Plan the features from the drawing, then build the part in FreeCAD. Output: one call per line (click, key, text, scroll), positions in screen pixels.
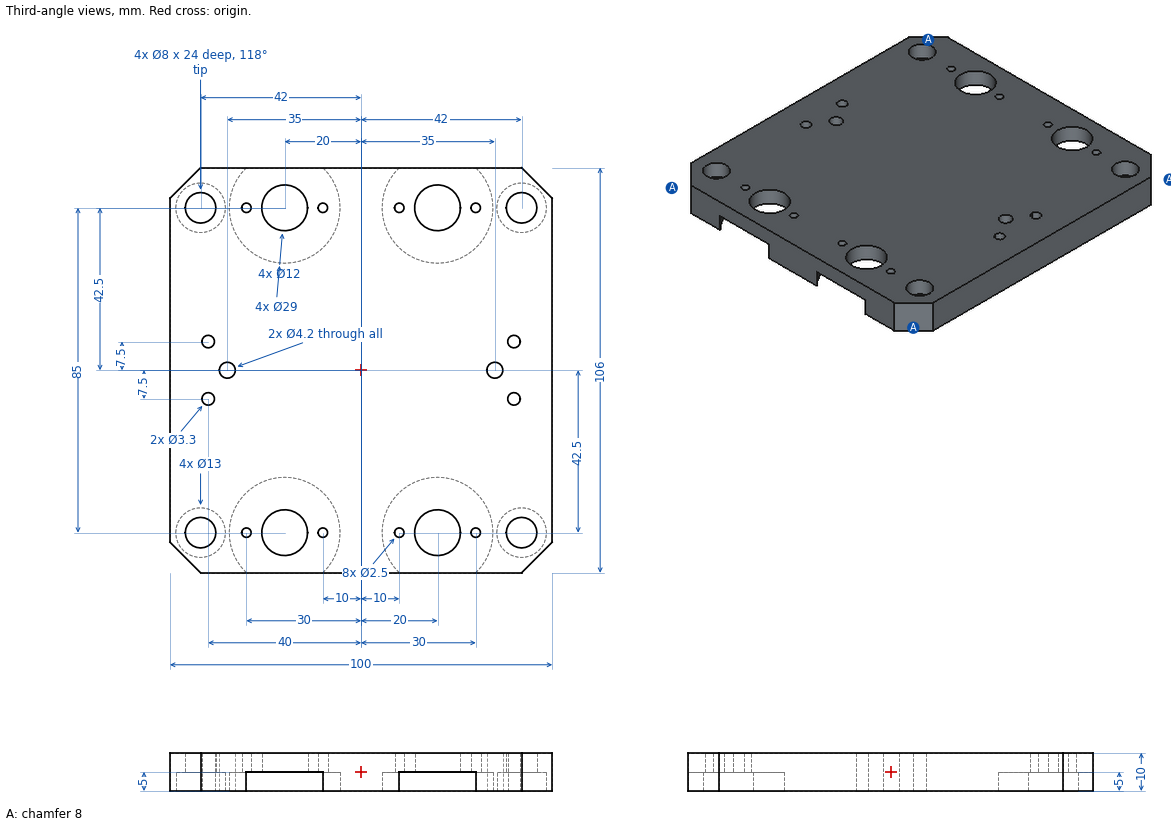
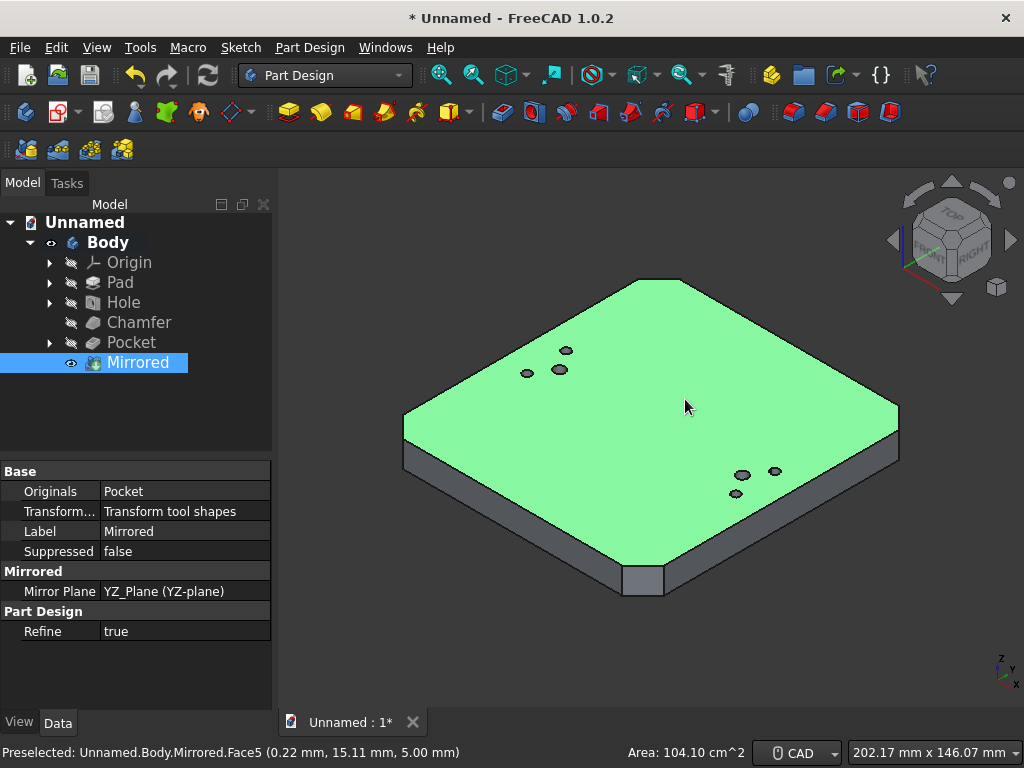
click(58, 112)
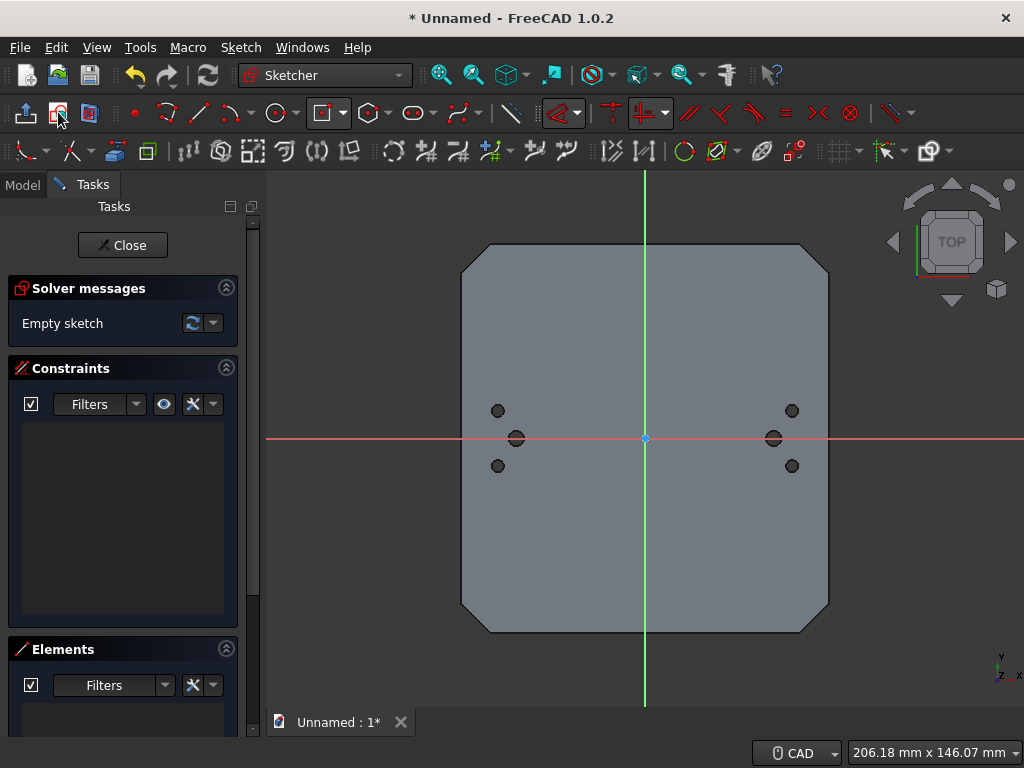
click(276, 114)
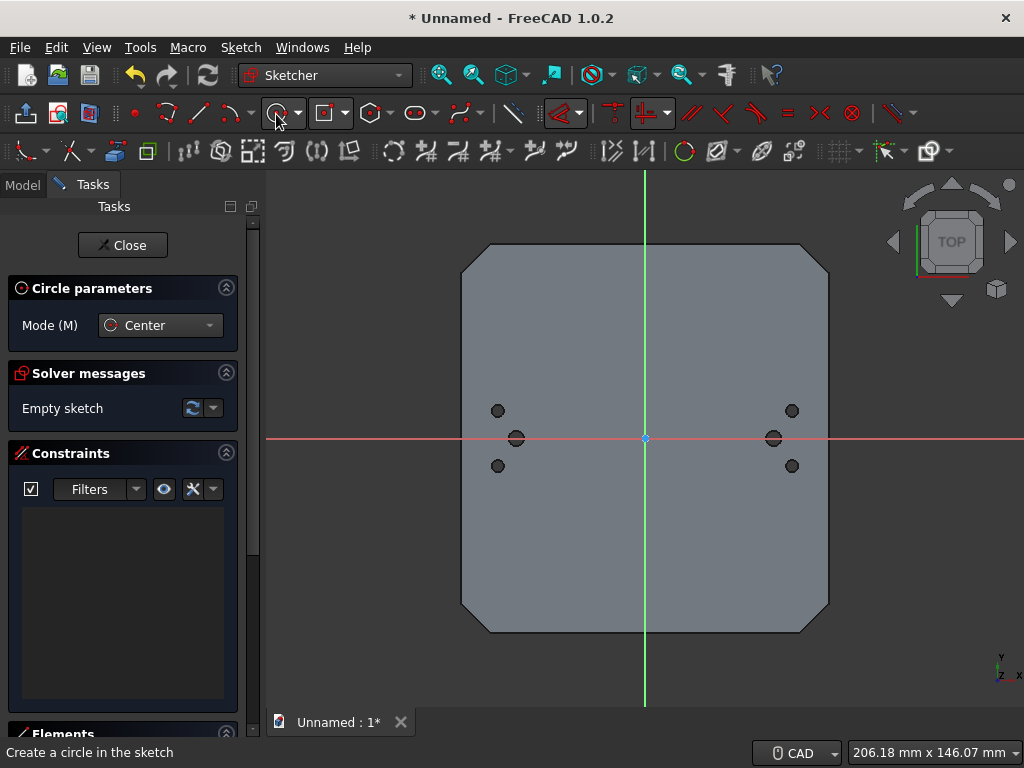
click(571, 282)
move(587, 267)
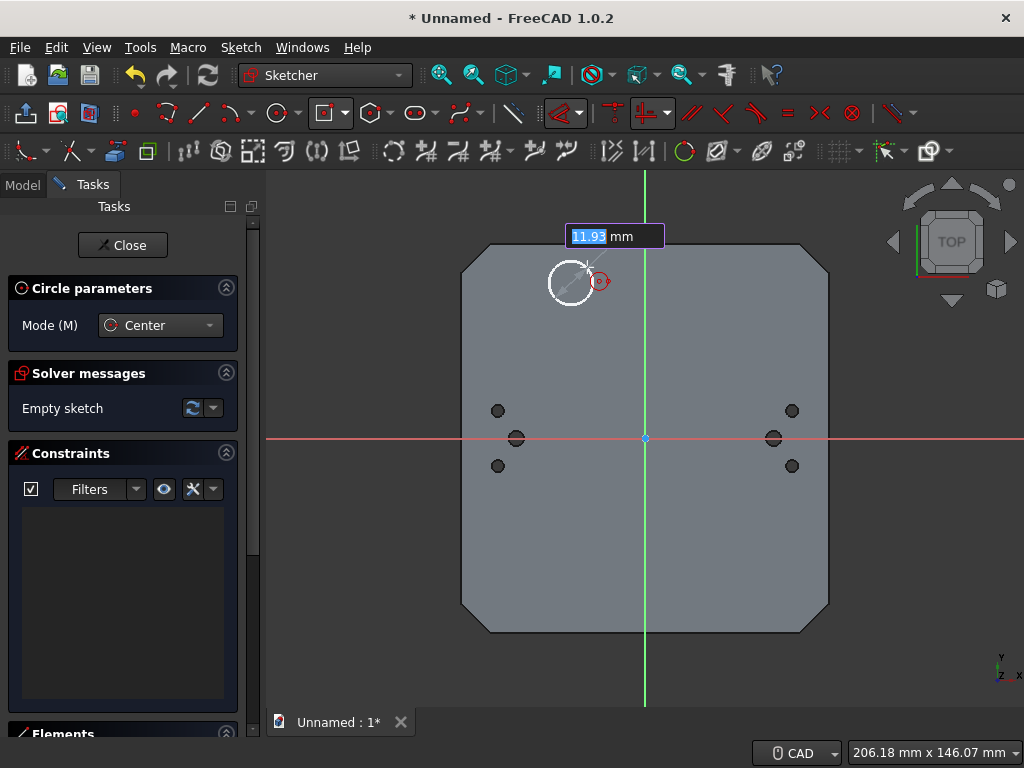
text(12)
key(Return)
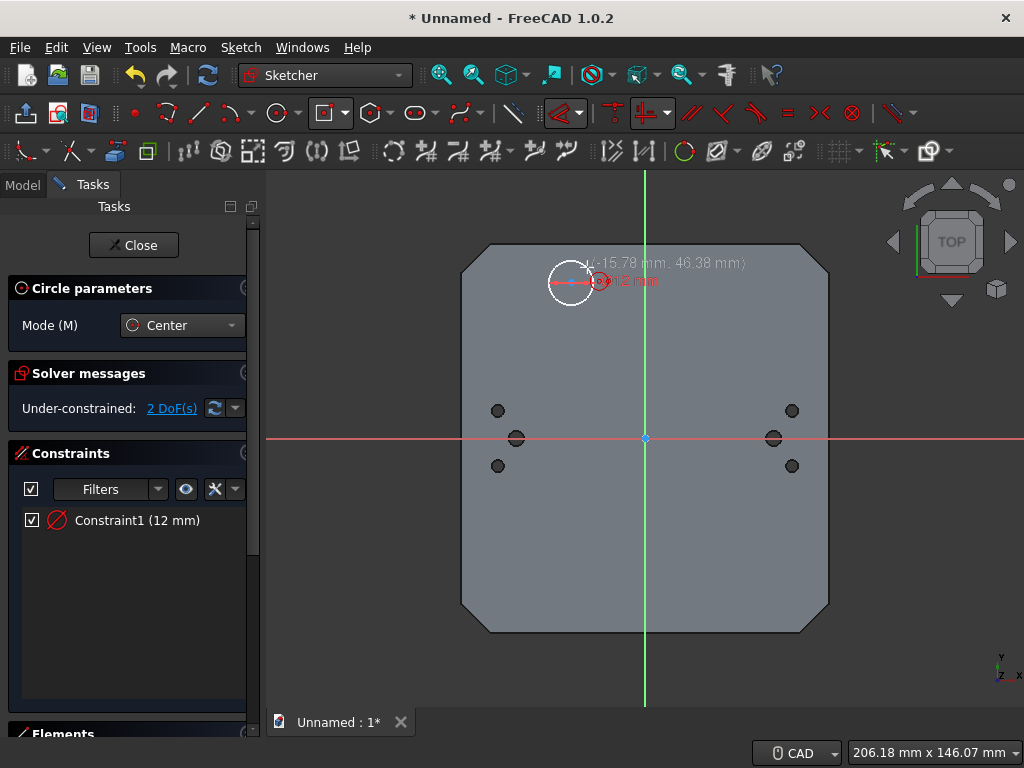
click(571, 595)
move(587, 579)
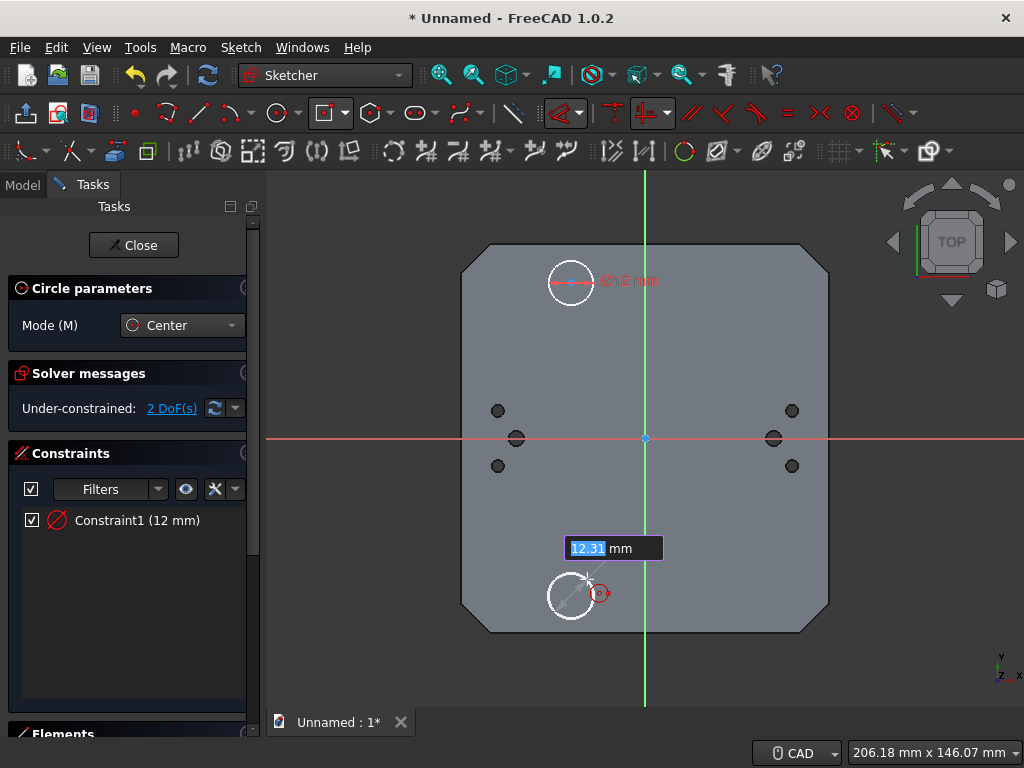
text(12)
key(Return)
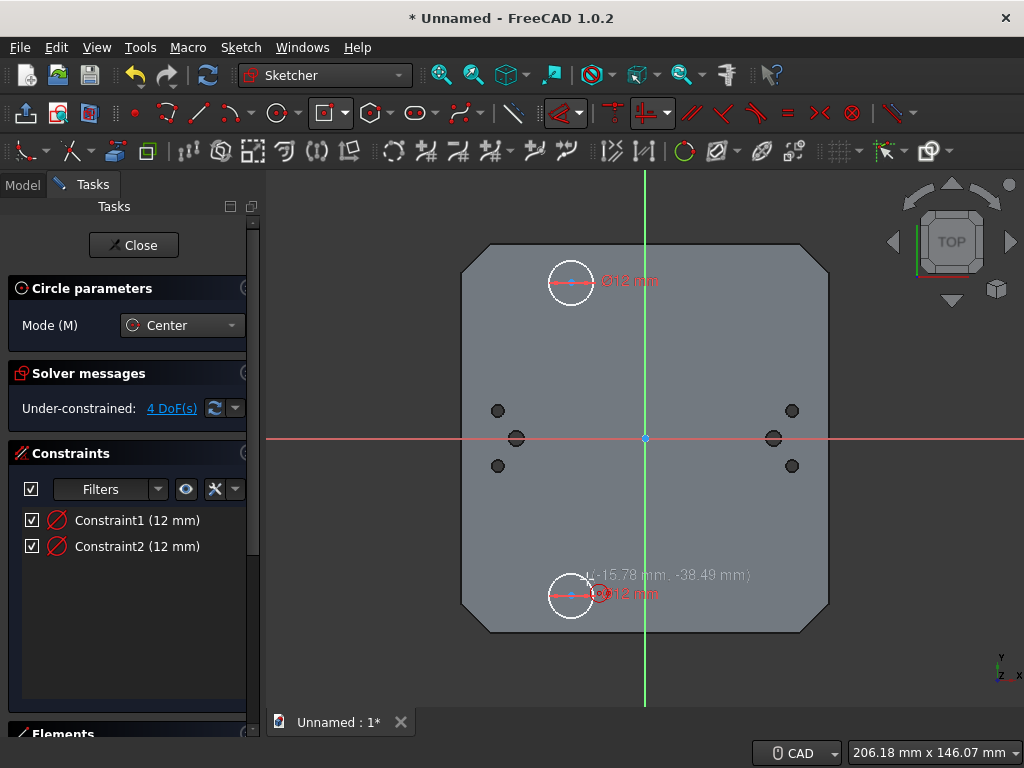
click(719, 595)
move(734, 579)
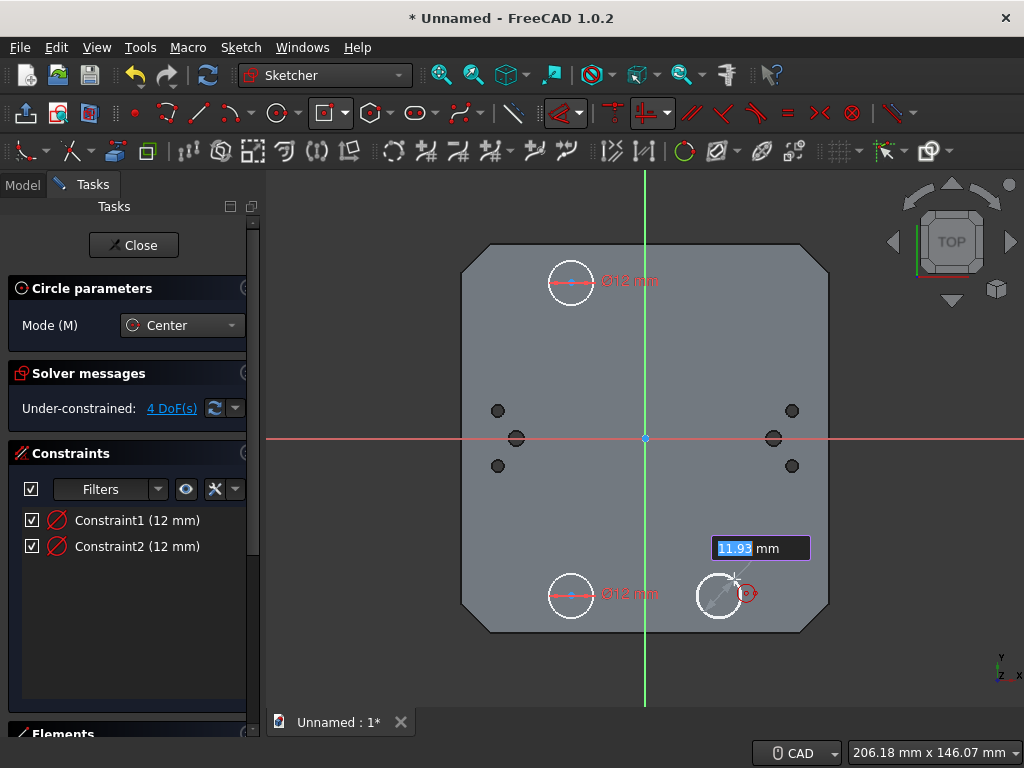
text(12)
key(Return)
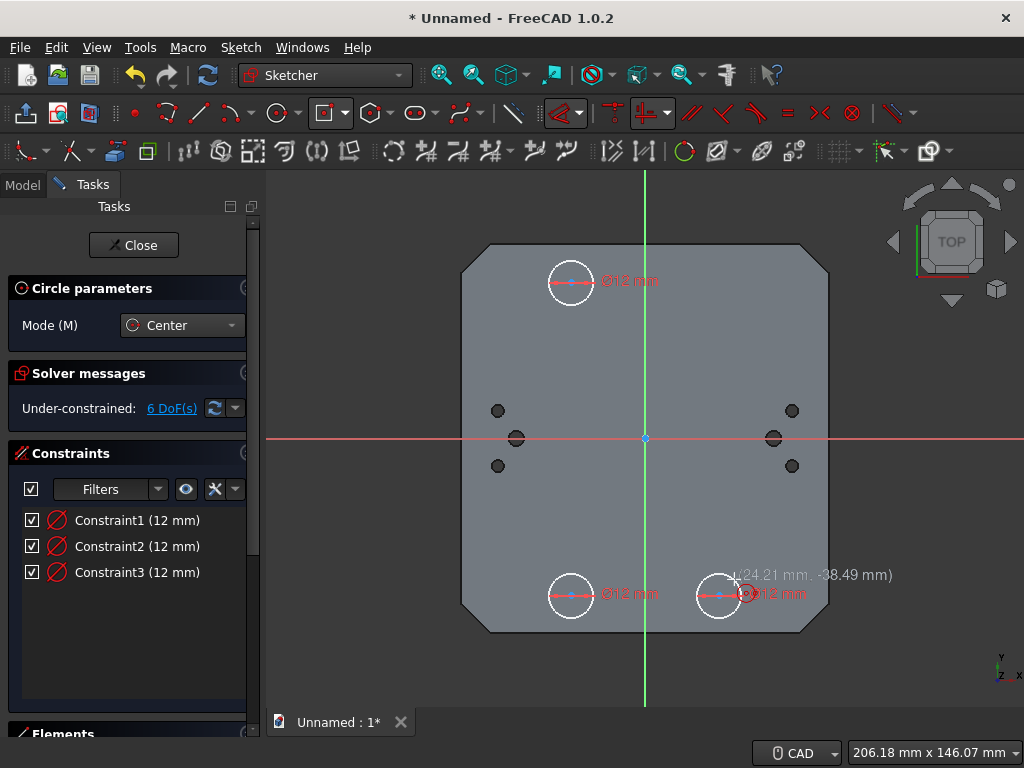
click(719, 282)
move(734, 267)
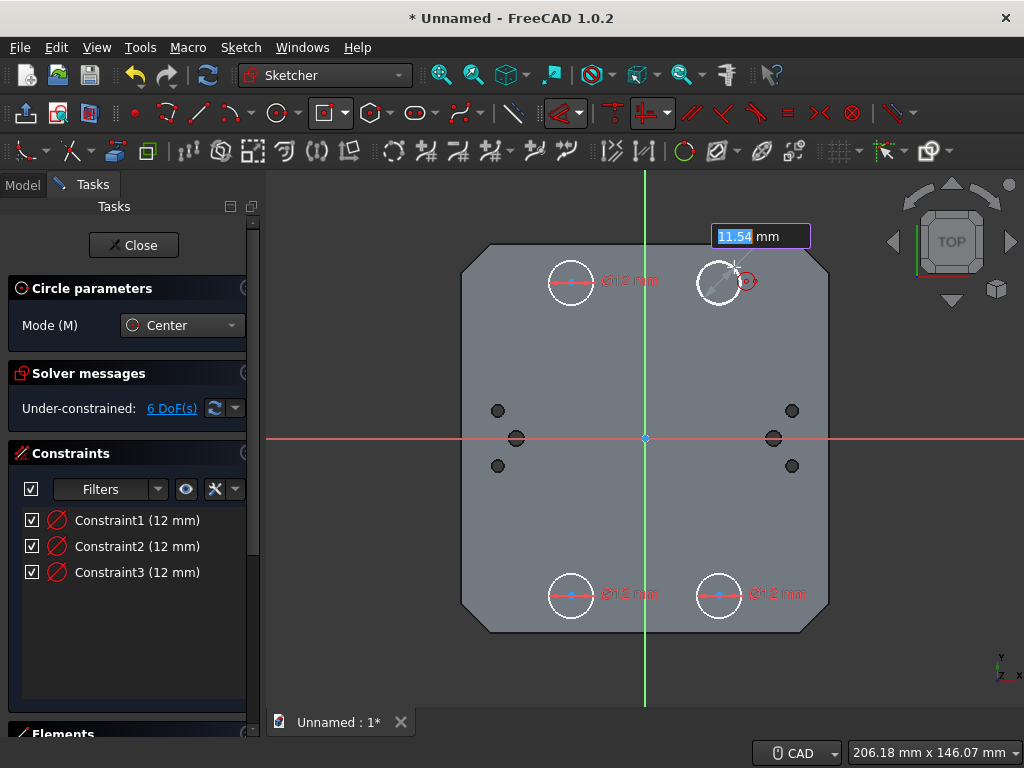
text(12)
key(Return)
key(Escape)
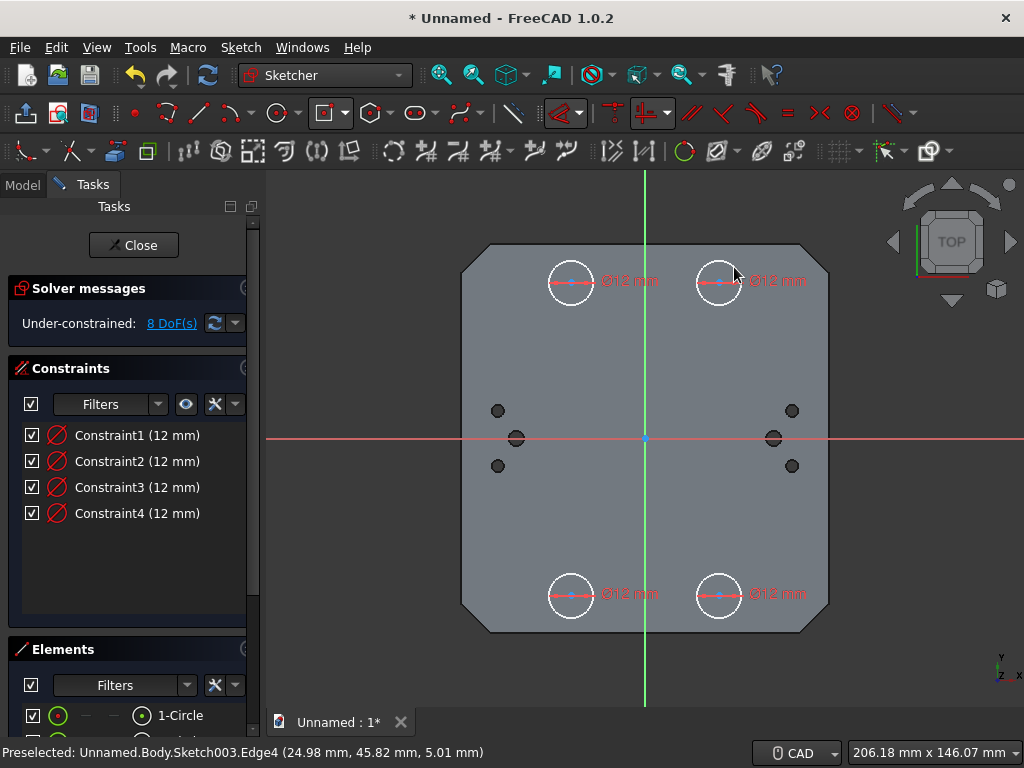
click(571, 283)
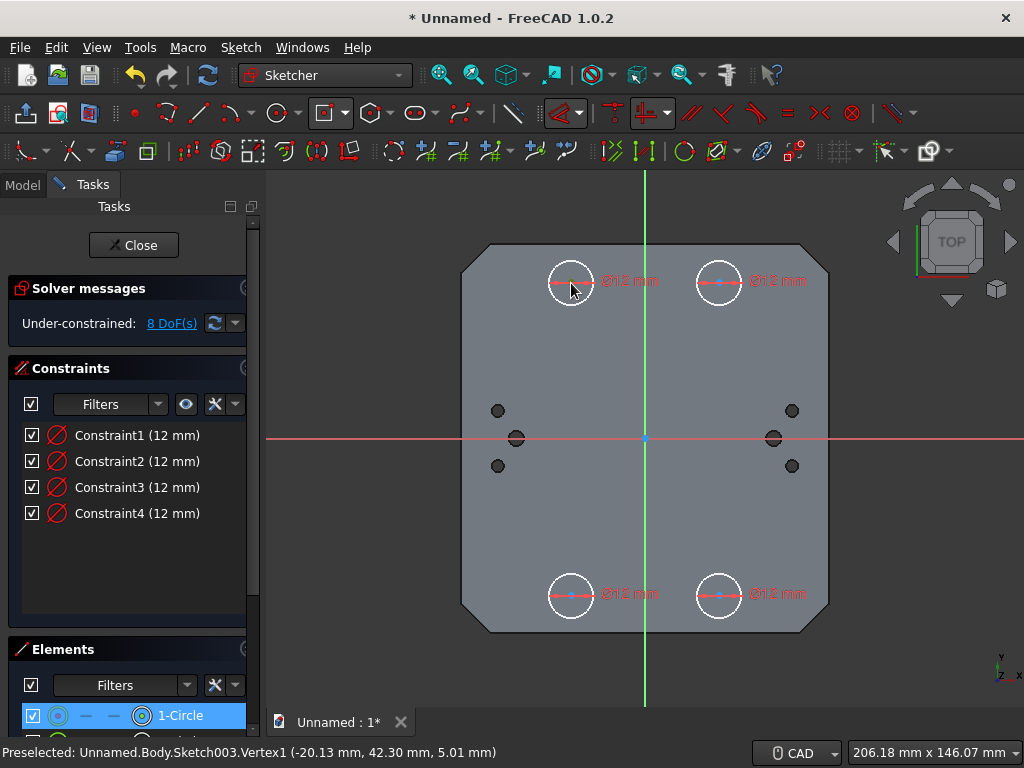
click(571, 596)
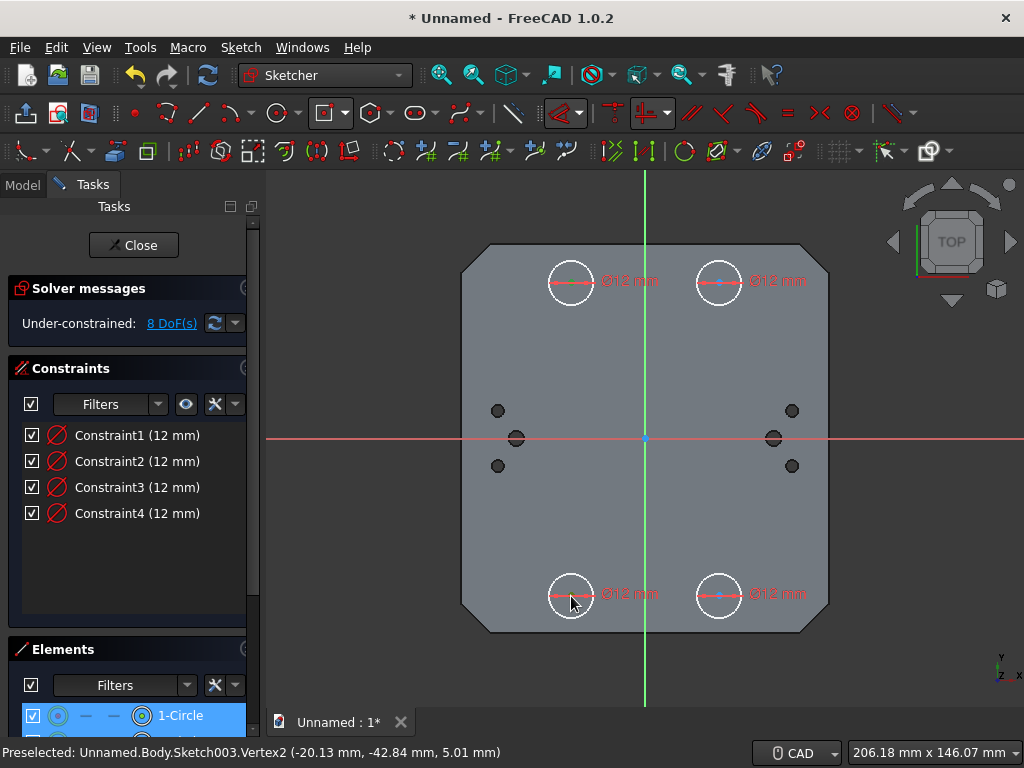
key(v)